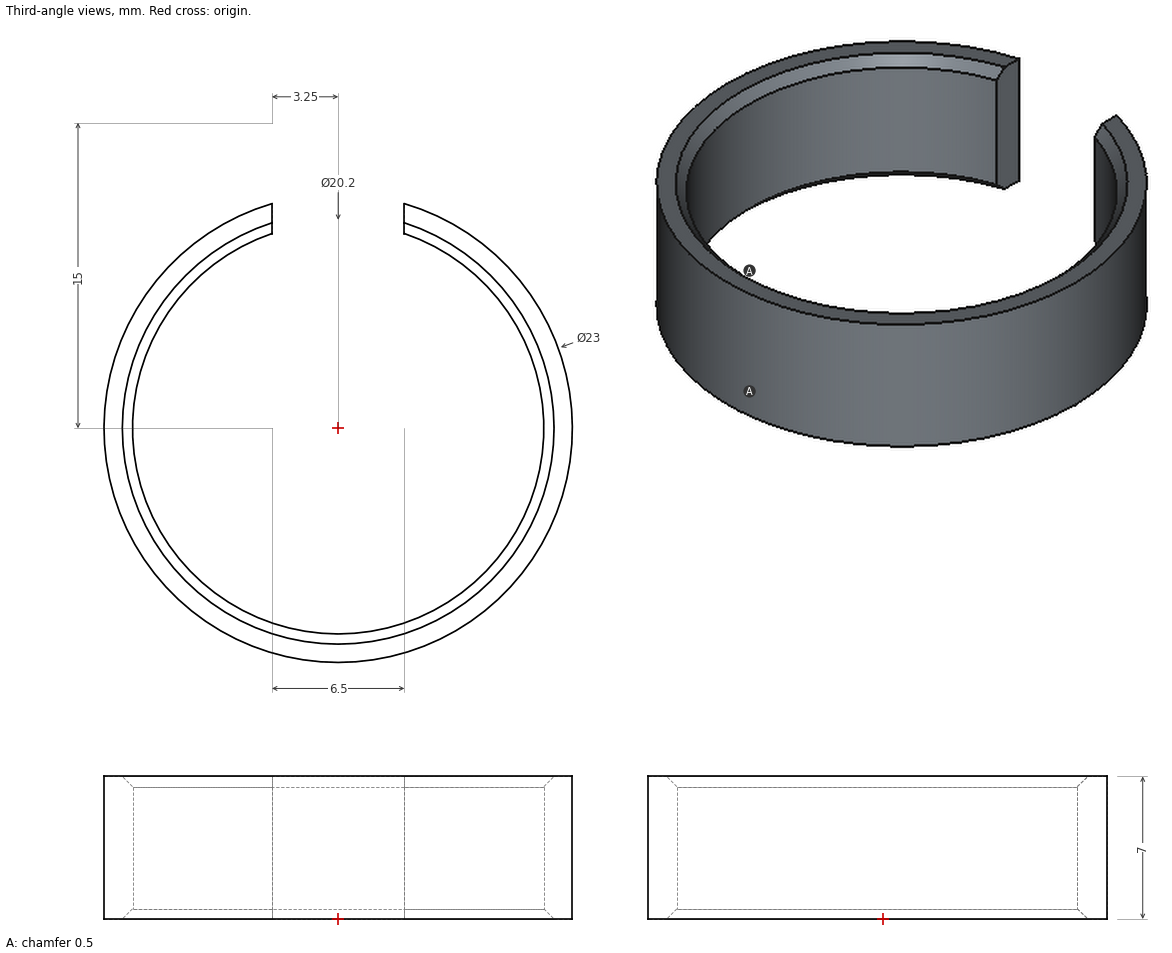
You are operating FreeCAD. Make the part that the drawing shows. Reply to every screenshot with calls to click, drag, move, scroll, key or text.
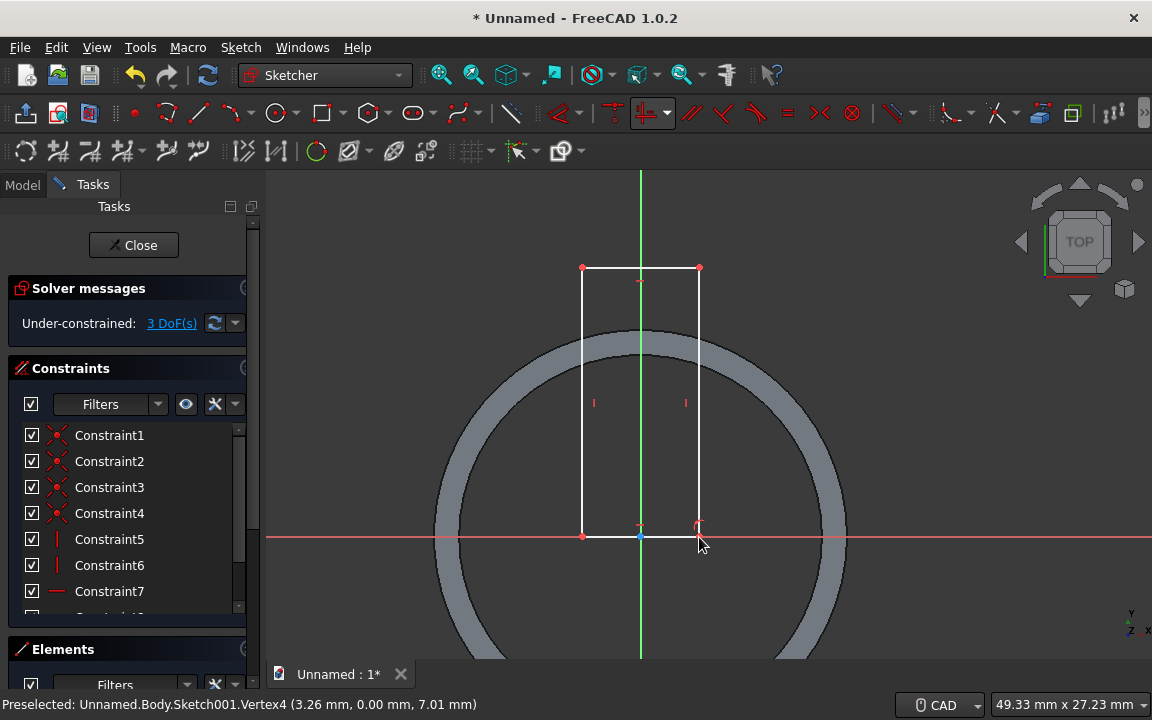
click(558, 114)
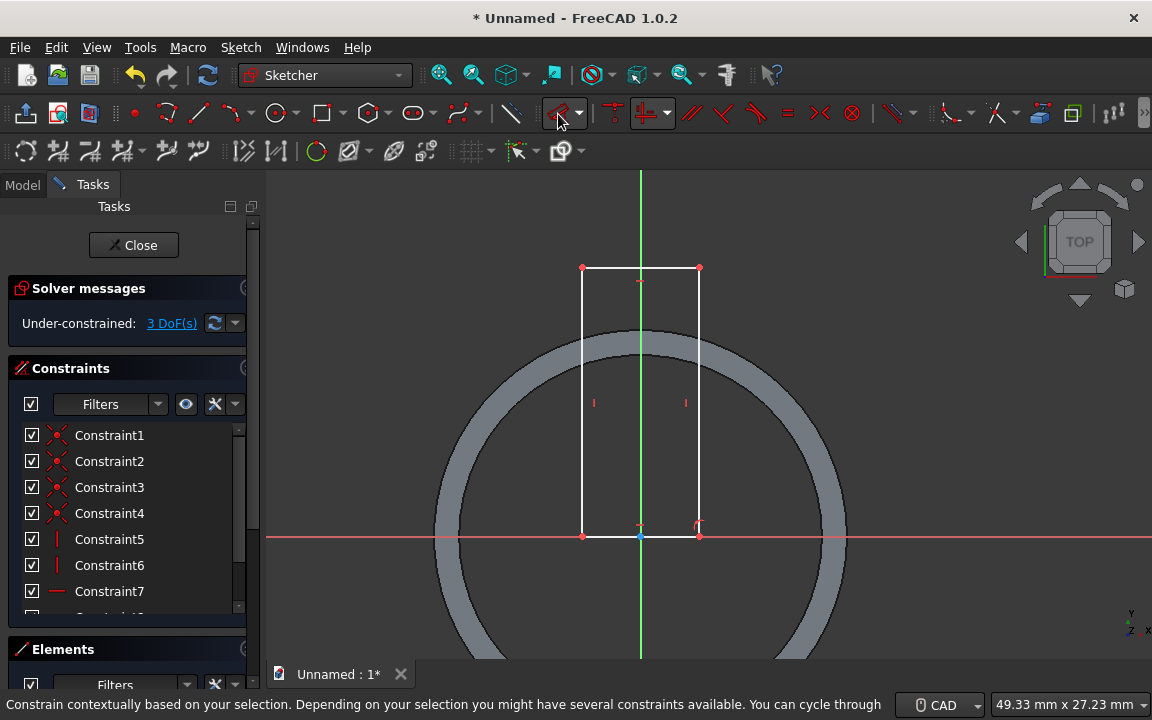
click(582, 349)
click(548, 402)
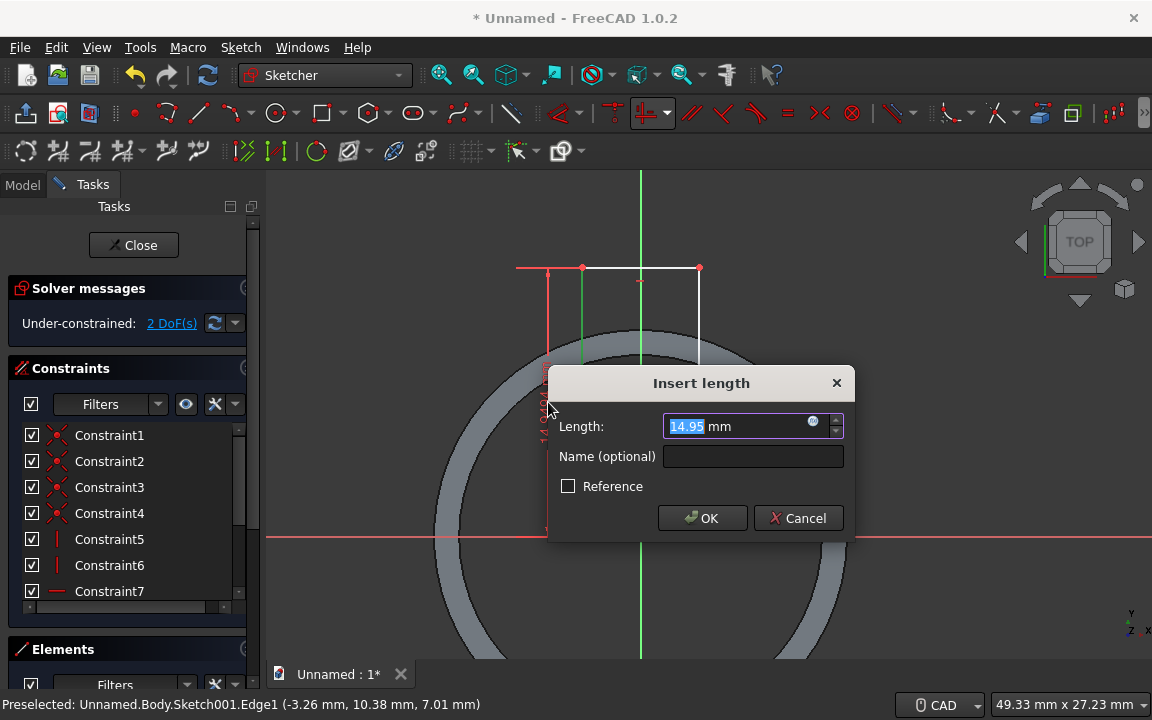
text(15)
key(Return)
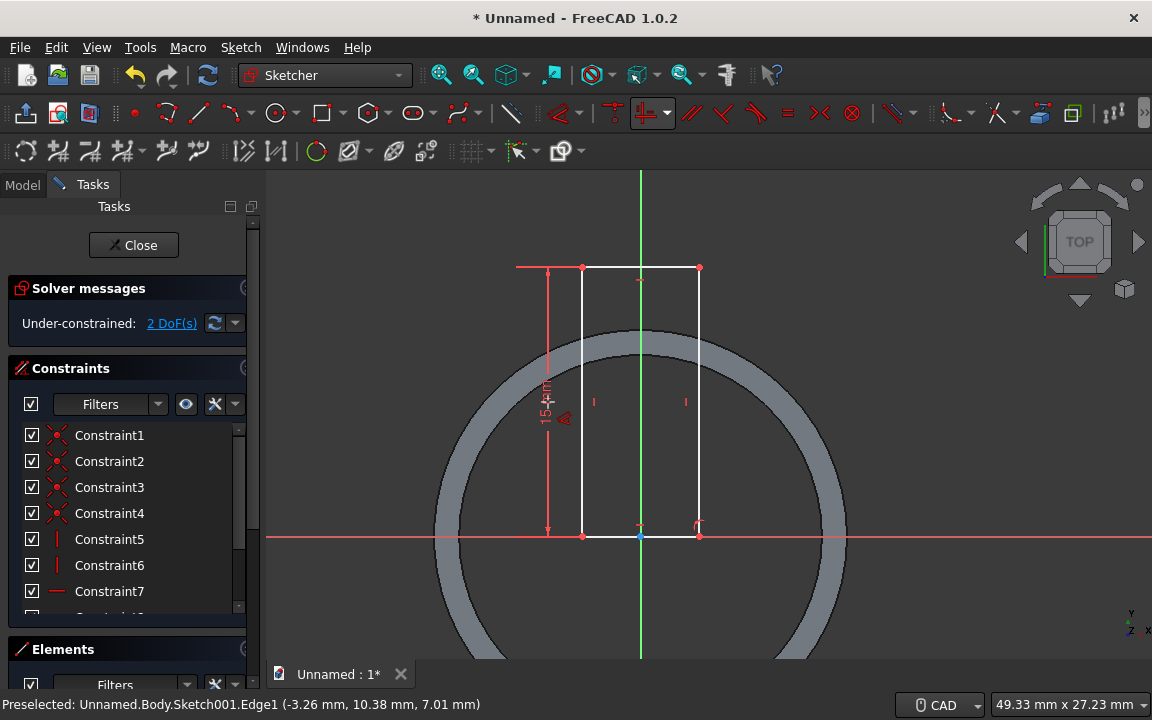
click(617, 537)
click(614, 571)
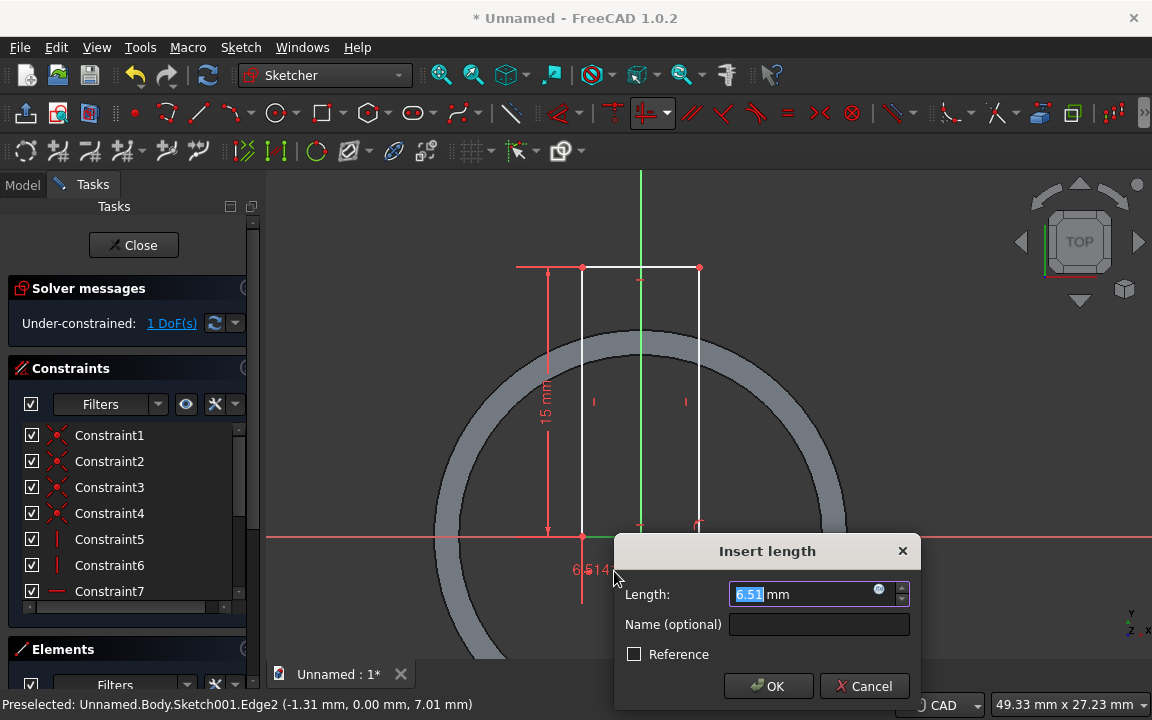
text(6.5)
key(Return)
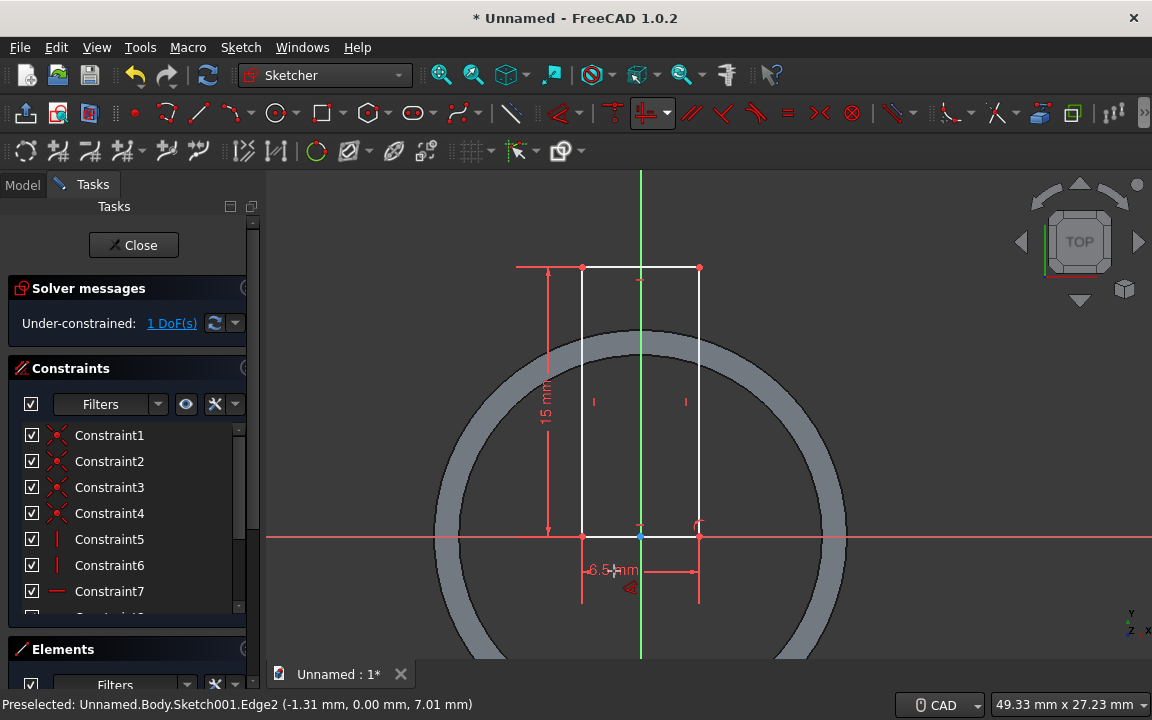
click(582, 267)
click(611, 233)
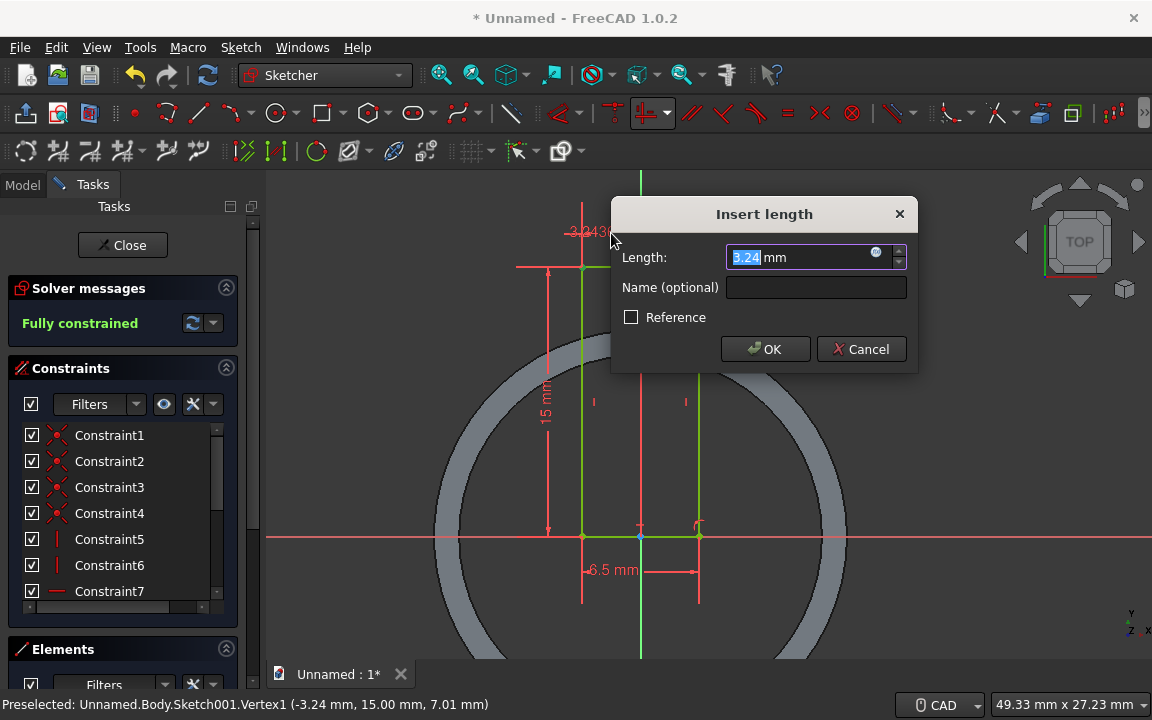
text(3.25)
key(Return)
key(Escape)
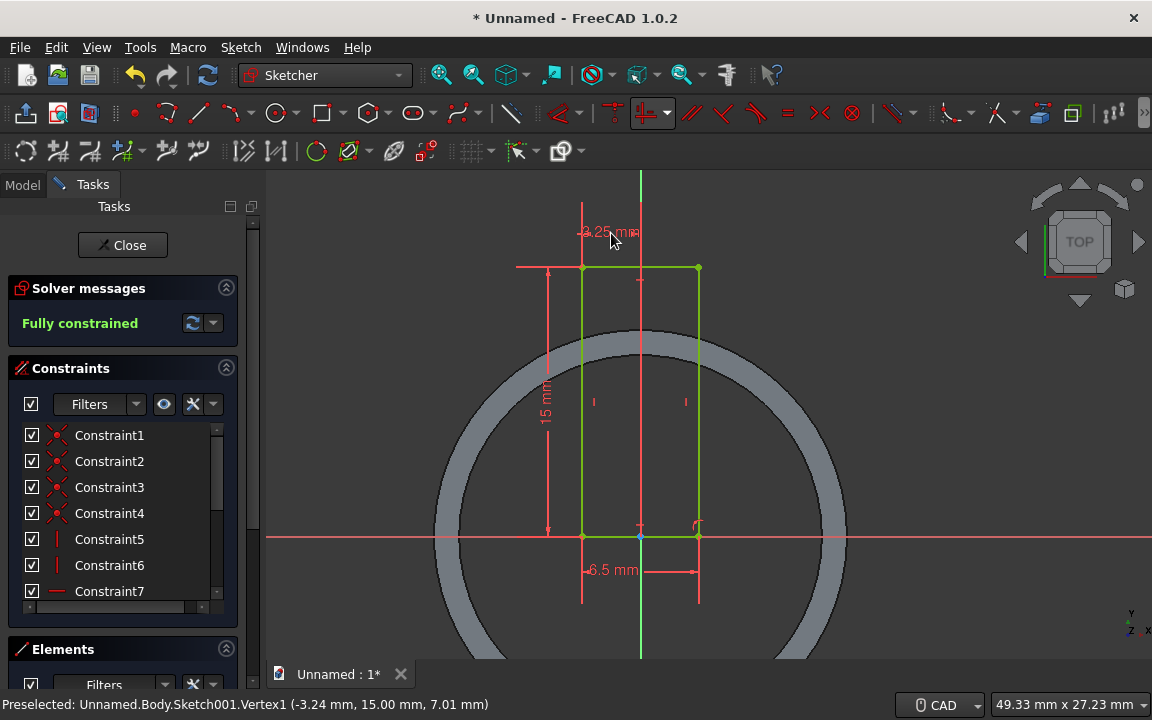
click(123, 245)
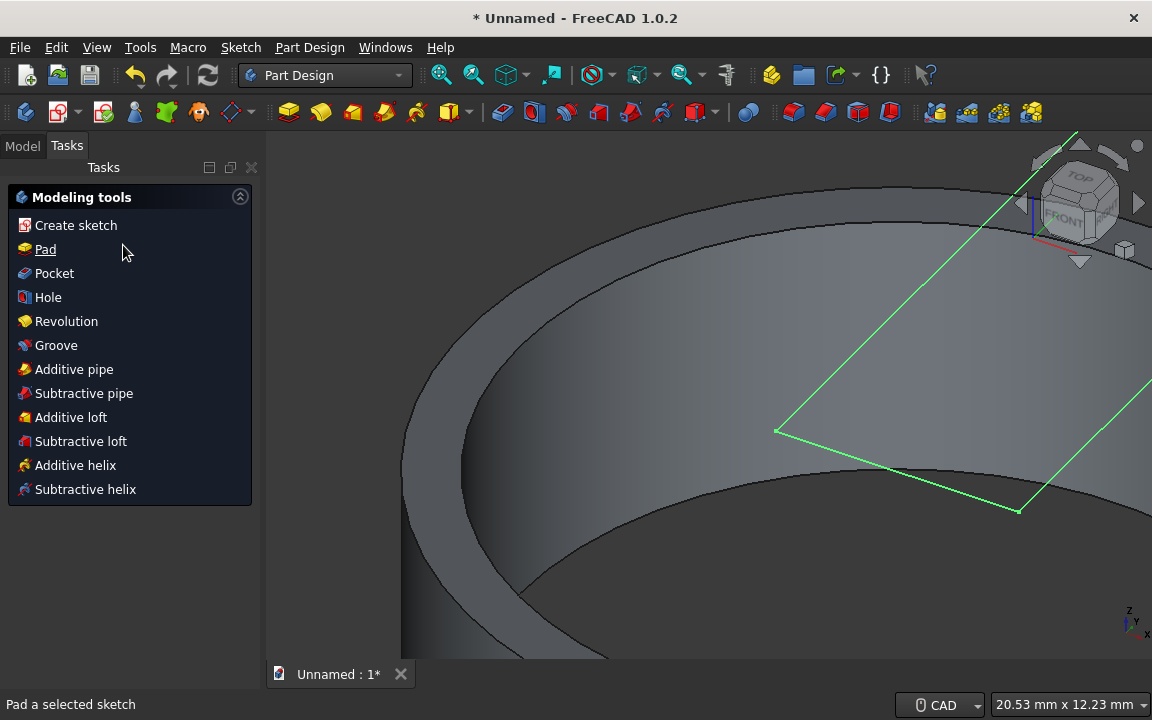
click(504, 112)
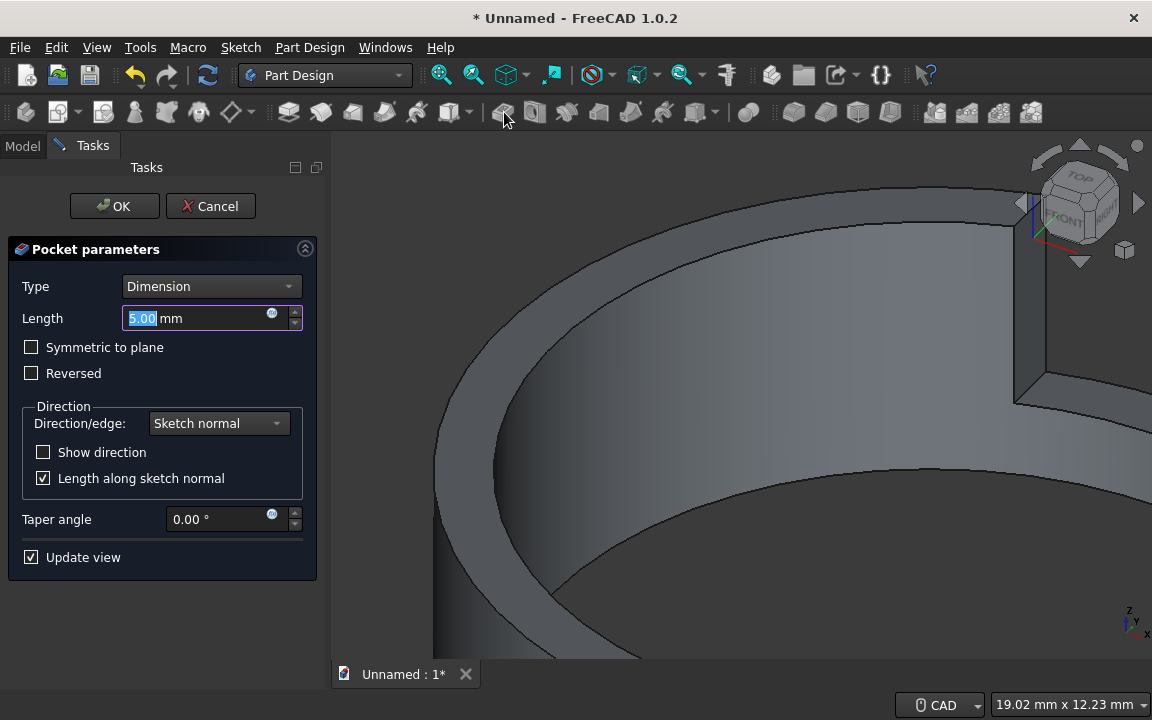
click(212, 286)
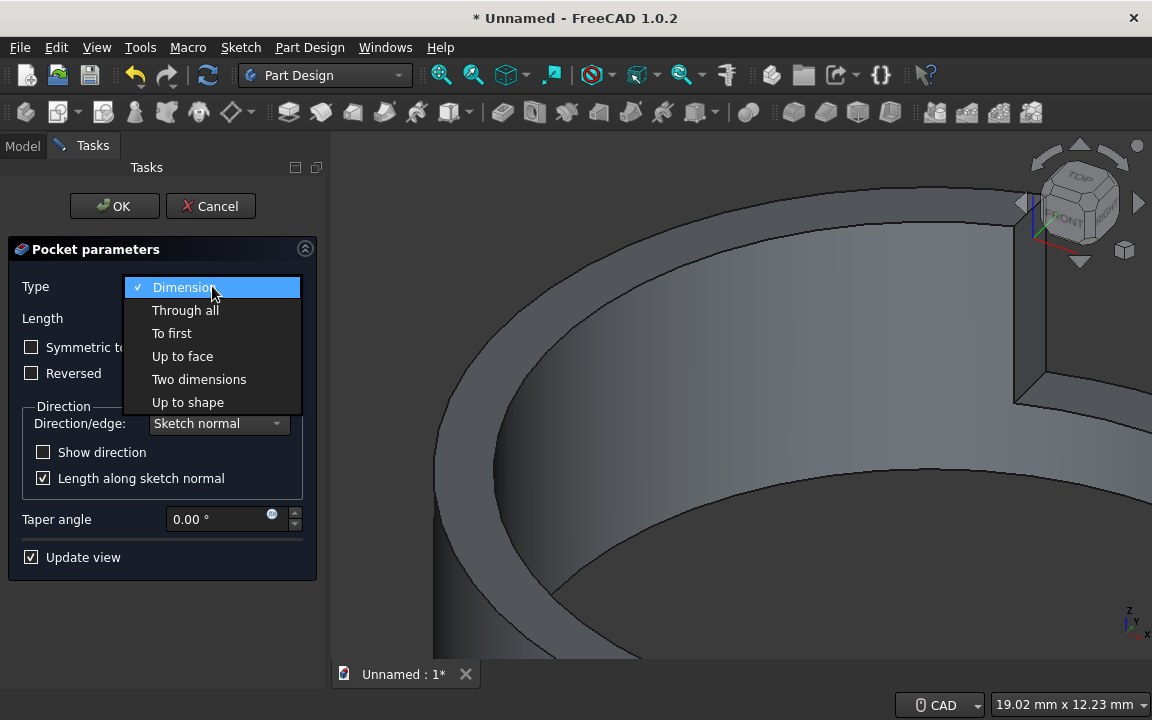
click(212, 310)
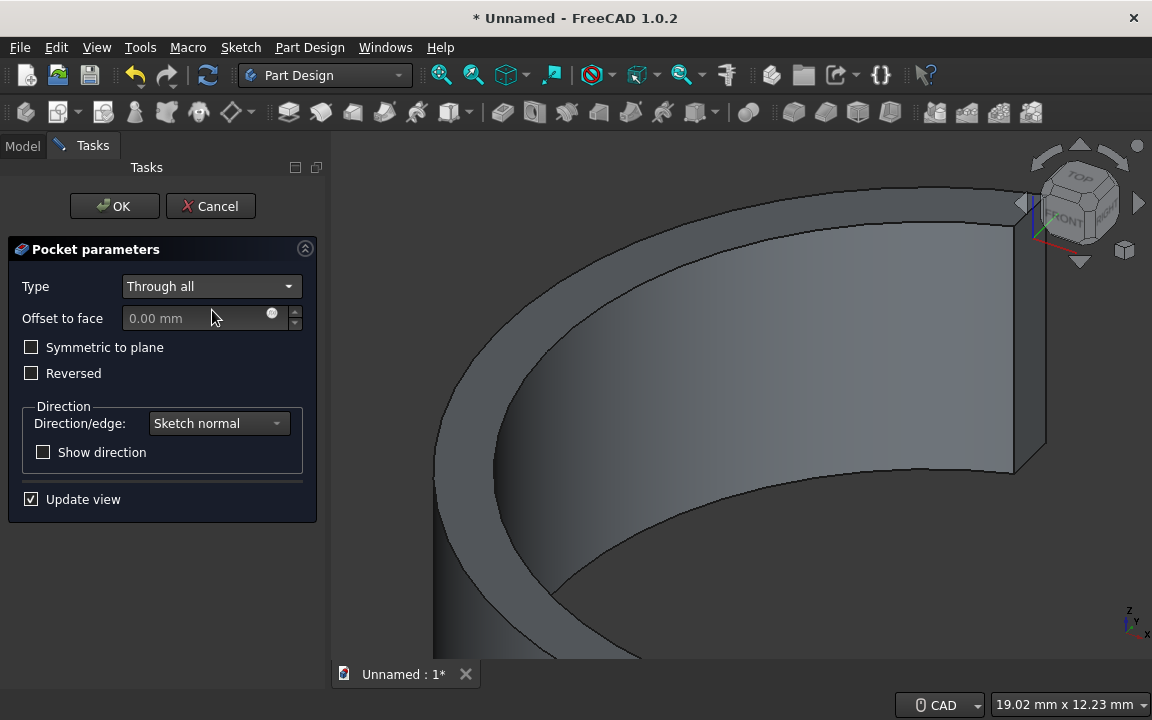
click(115, 206)